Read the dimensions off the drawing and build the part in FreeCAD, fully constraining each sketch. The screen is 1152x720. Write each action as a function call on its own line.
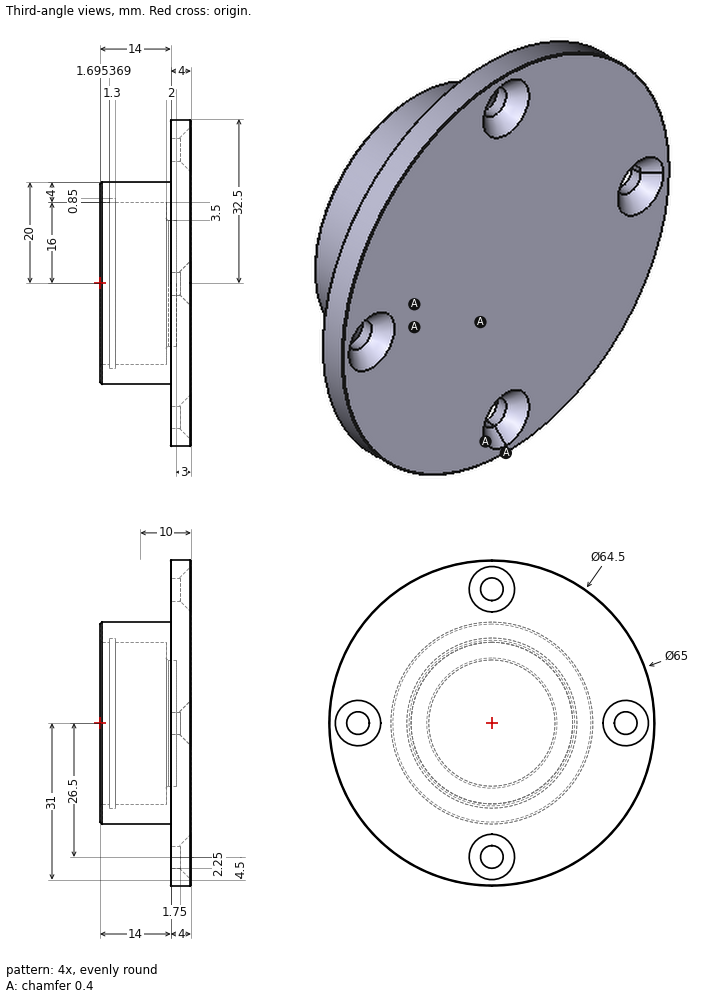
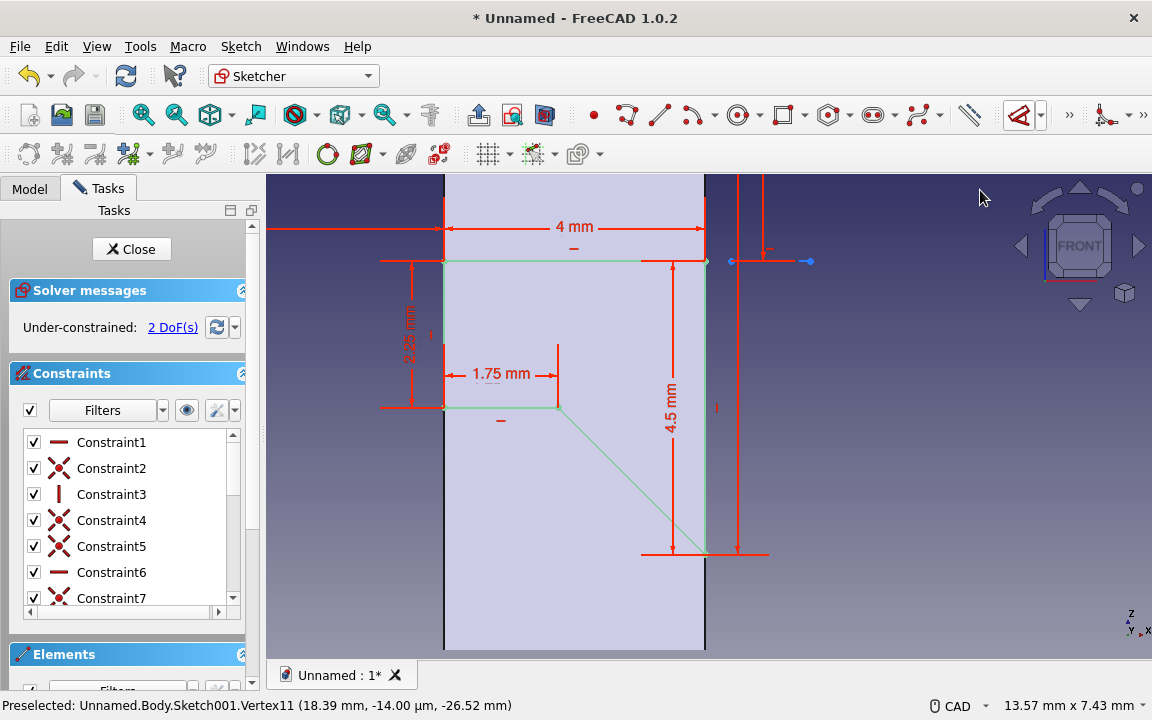
click(132, 249)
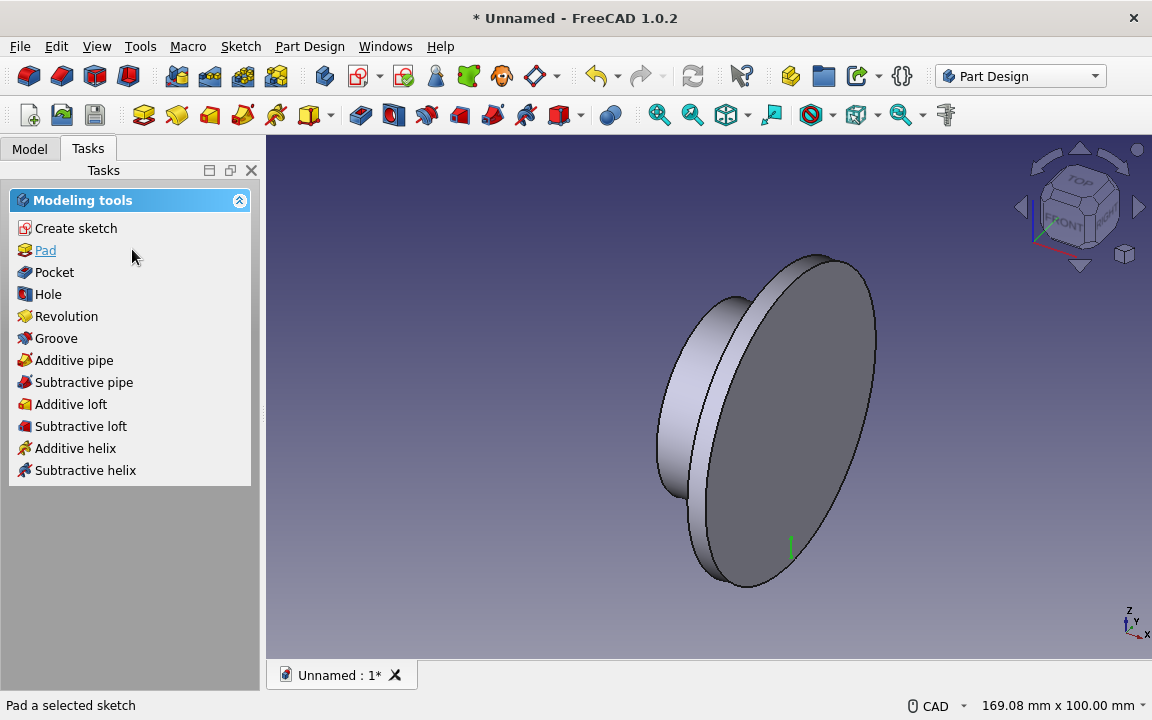
click(427, 116)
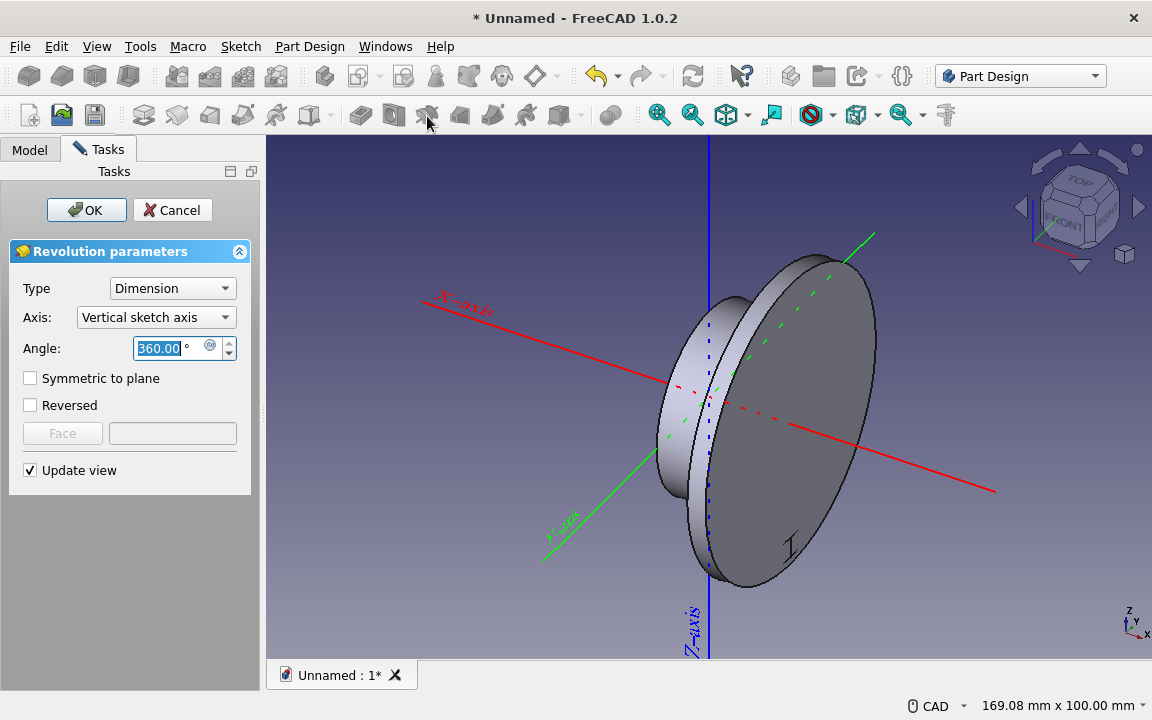
click(157, 318)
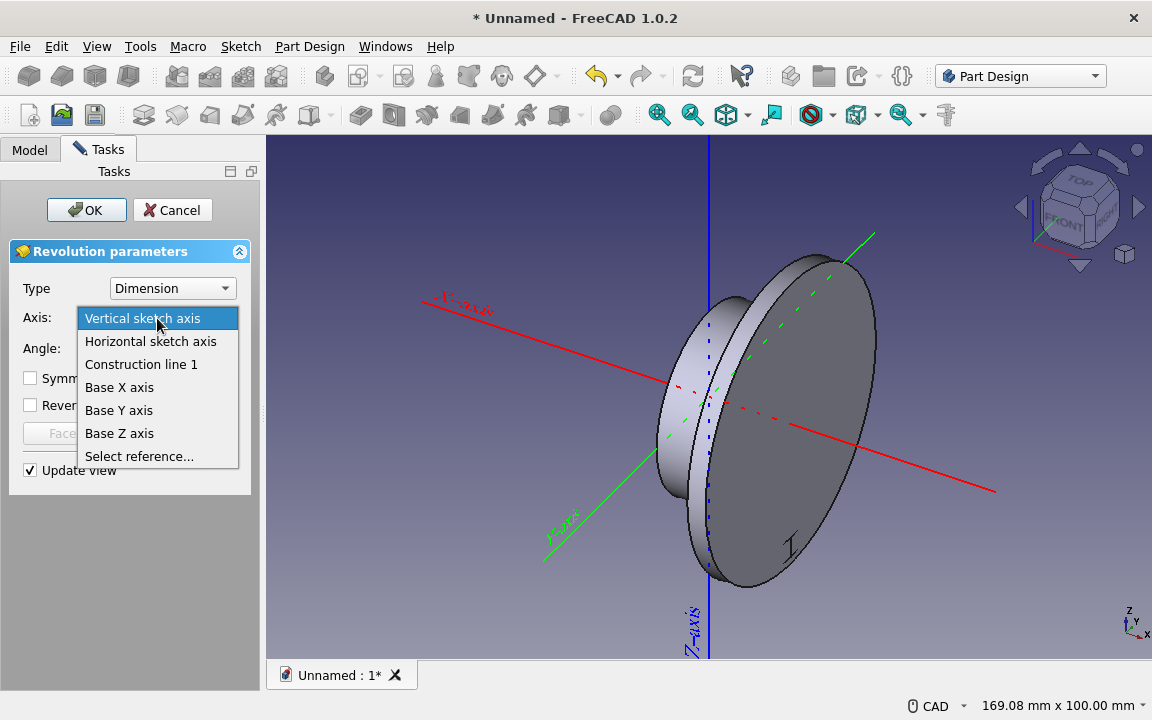
click(156, 364)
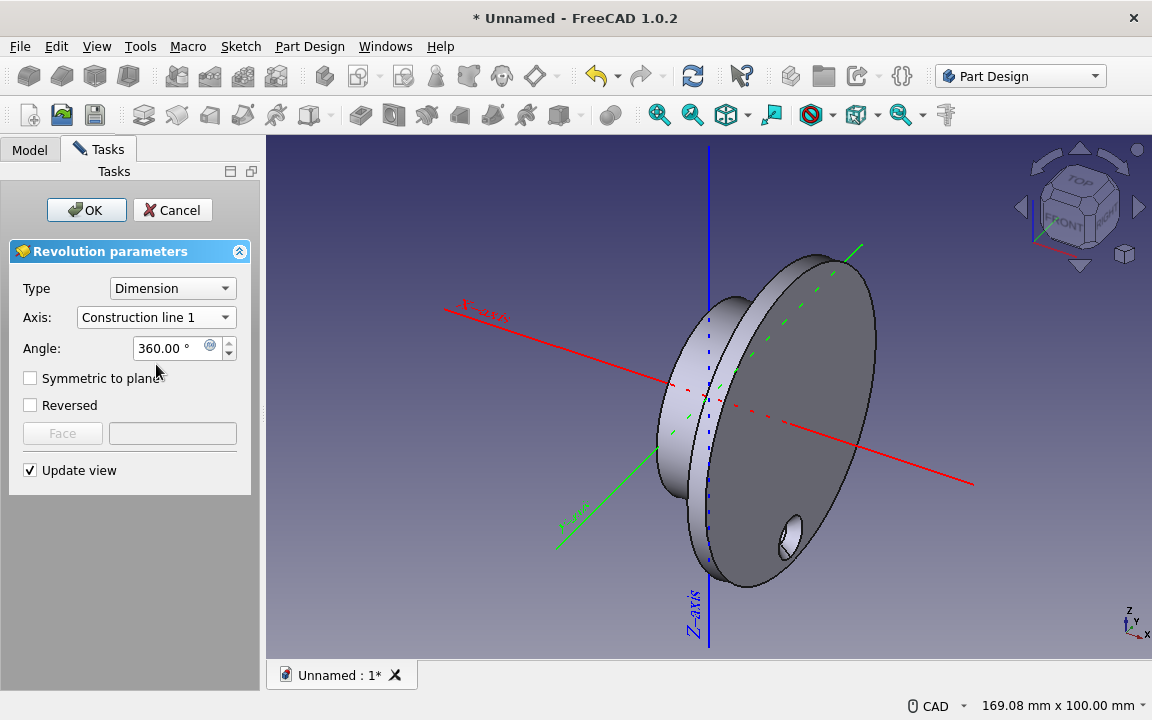
click(87, 210)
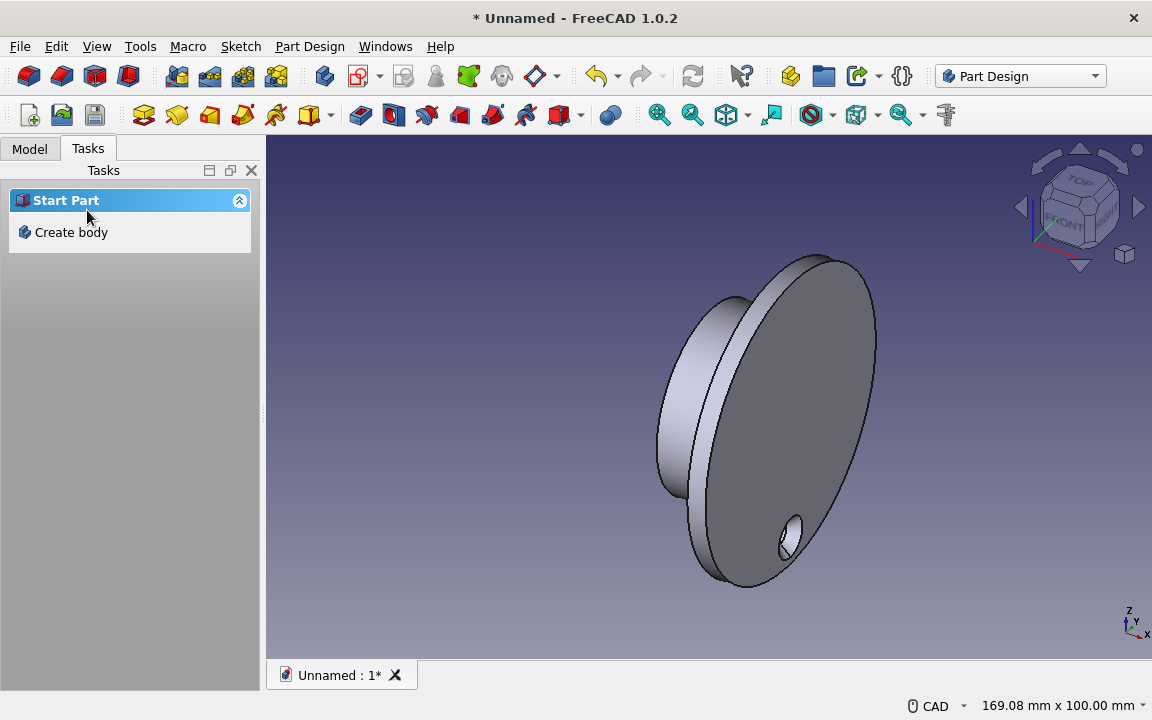
click(30, 148)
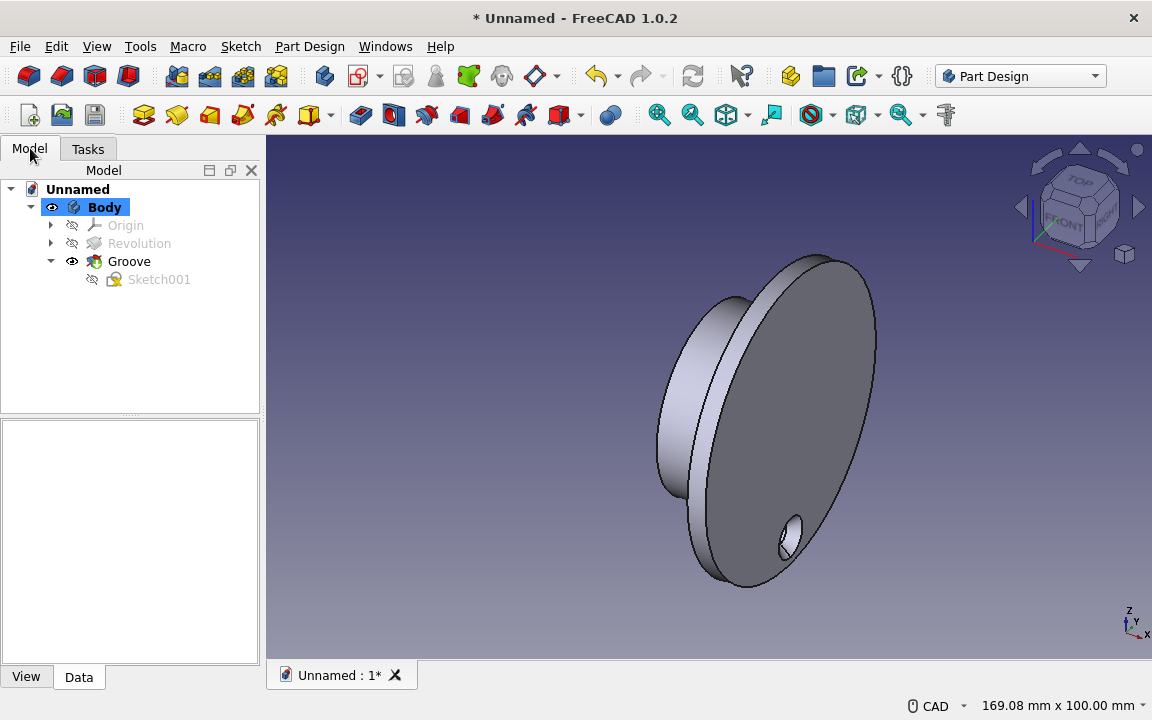
click(117, 261)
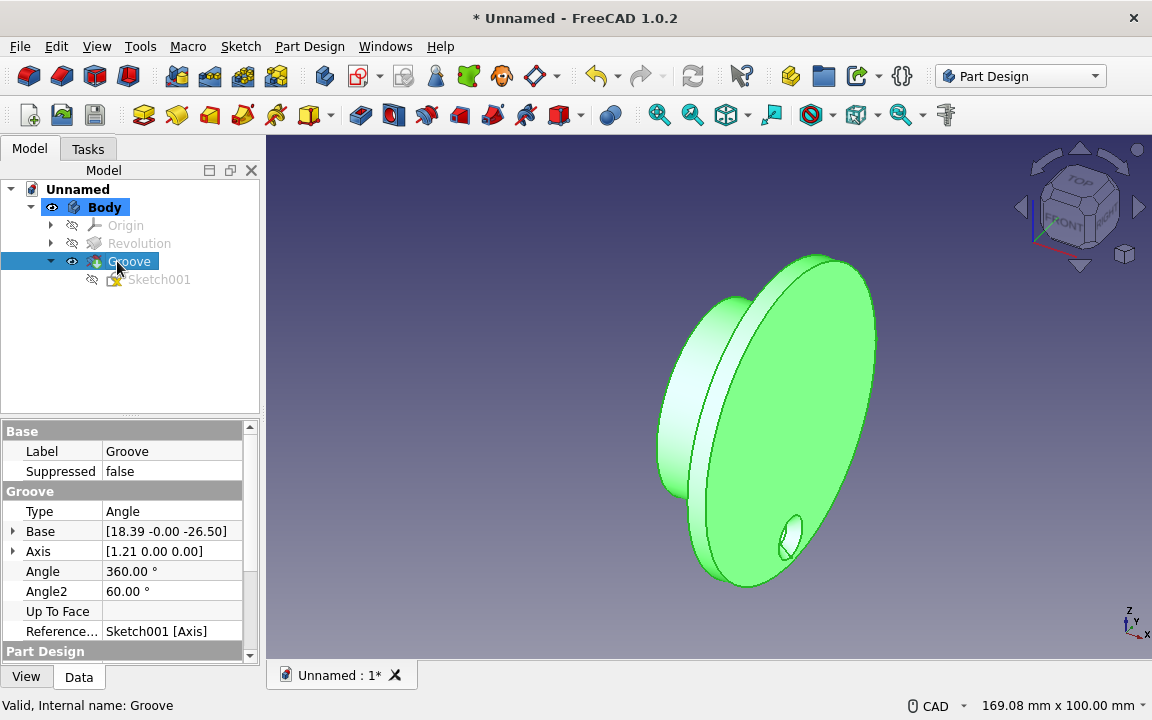
click(243, 76)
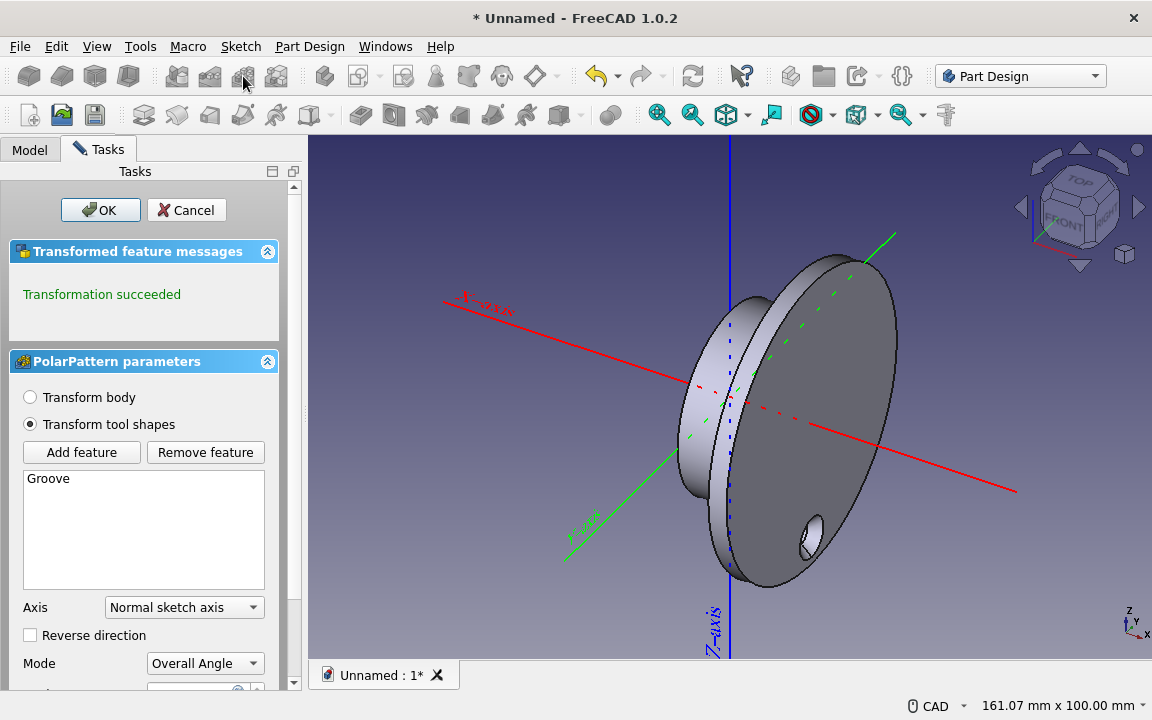
click(185, 608)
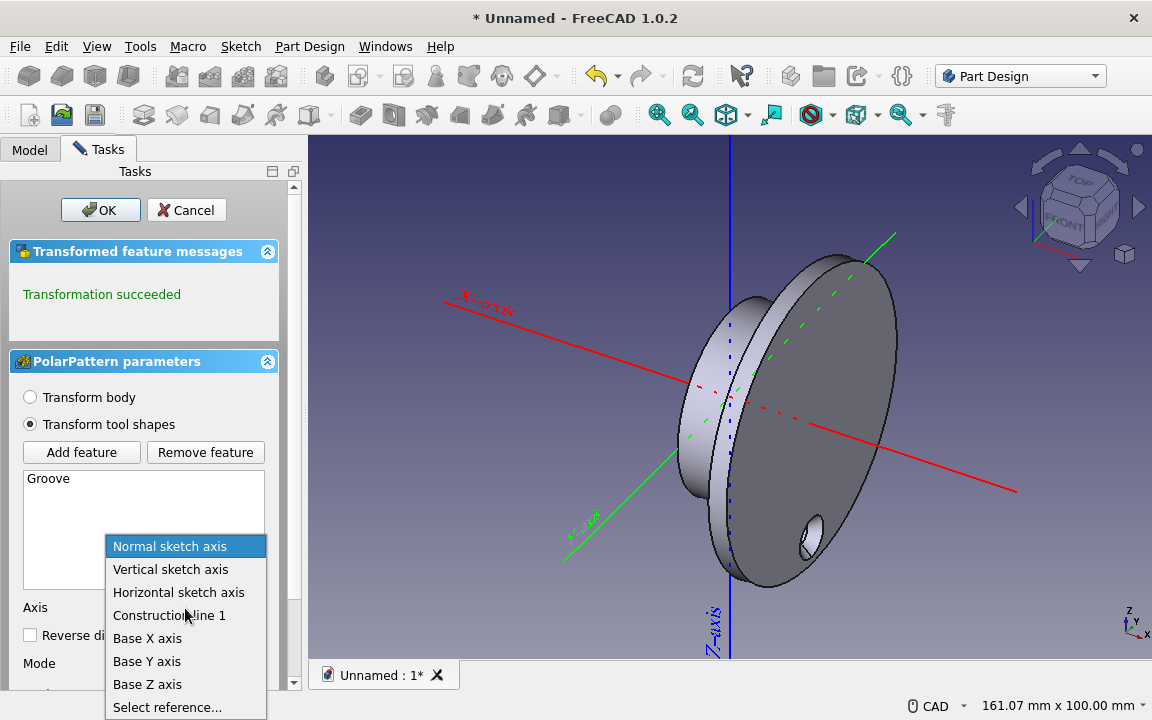
click(184, 638)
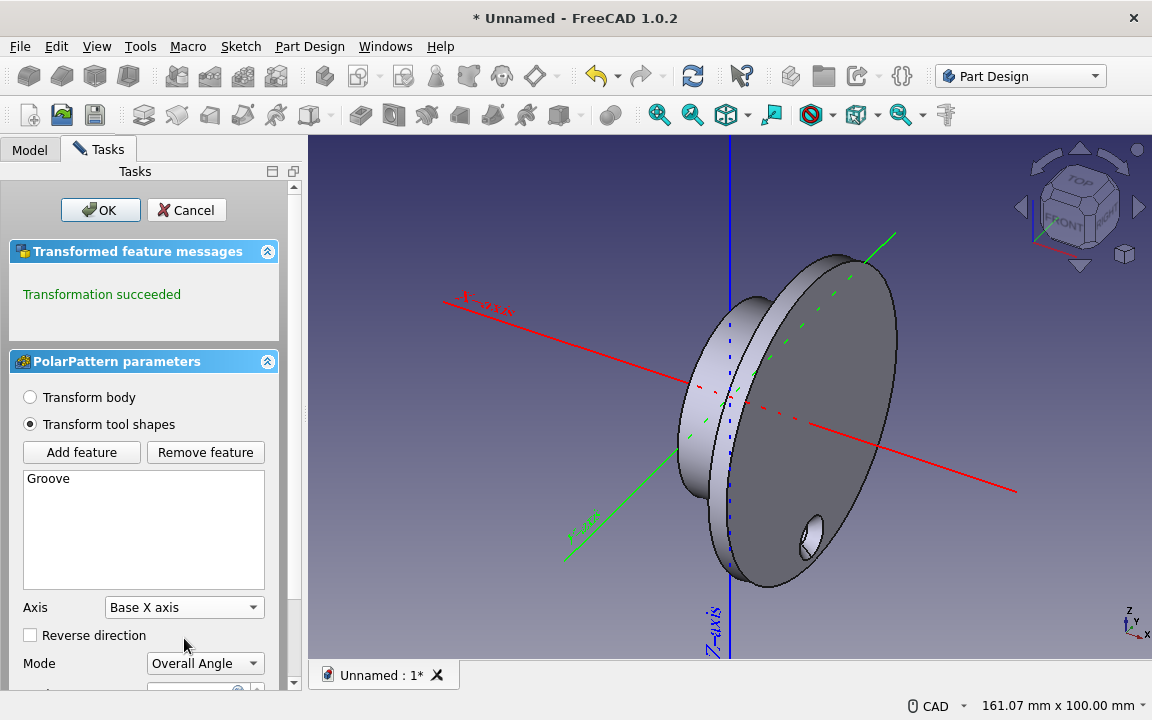
scroll(294, 436, down, 2)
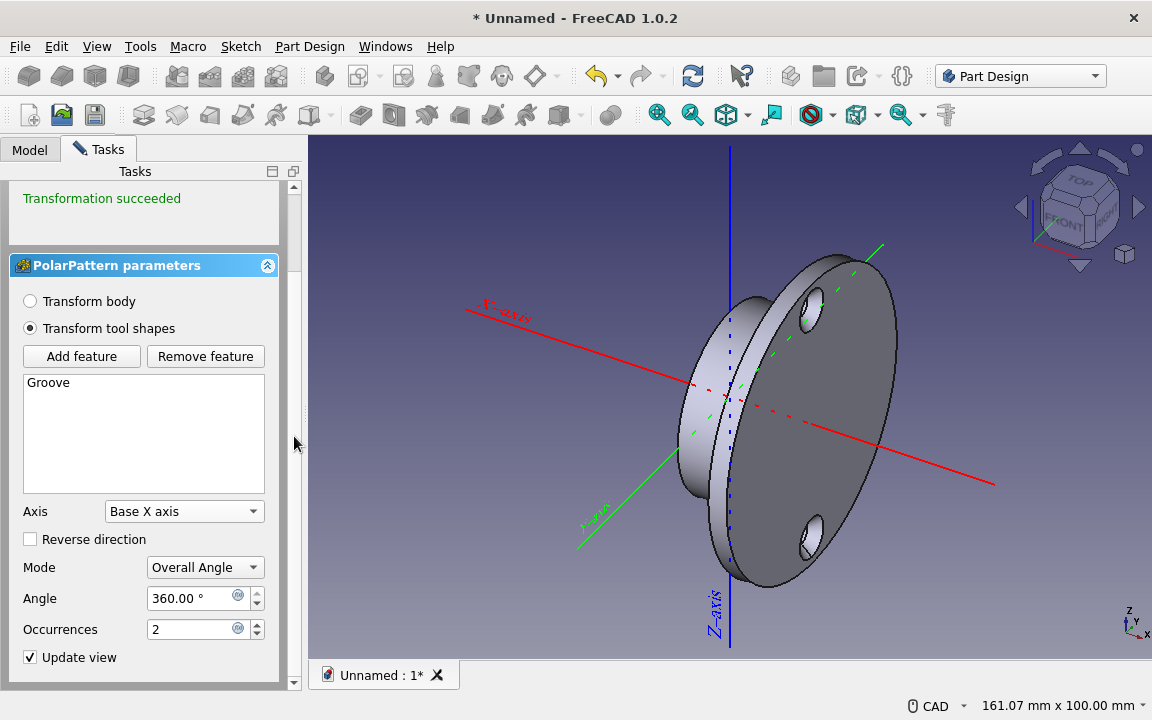
triple_click(199, 630)